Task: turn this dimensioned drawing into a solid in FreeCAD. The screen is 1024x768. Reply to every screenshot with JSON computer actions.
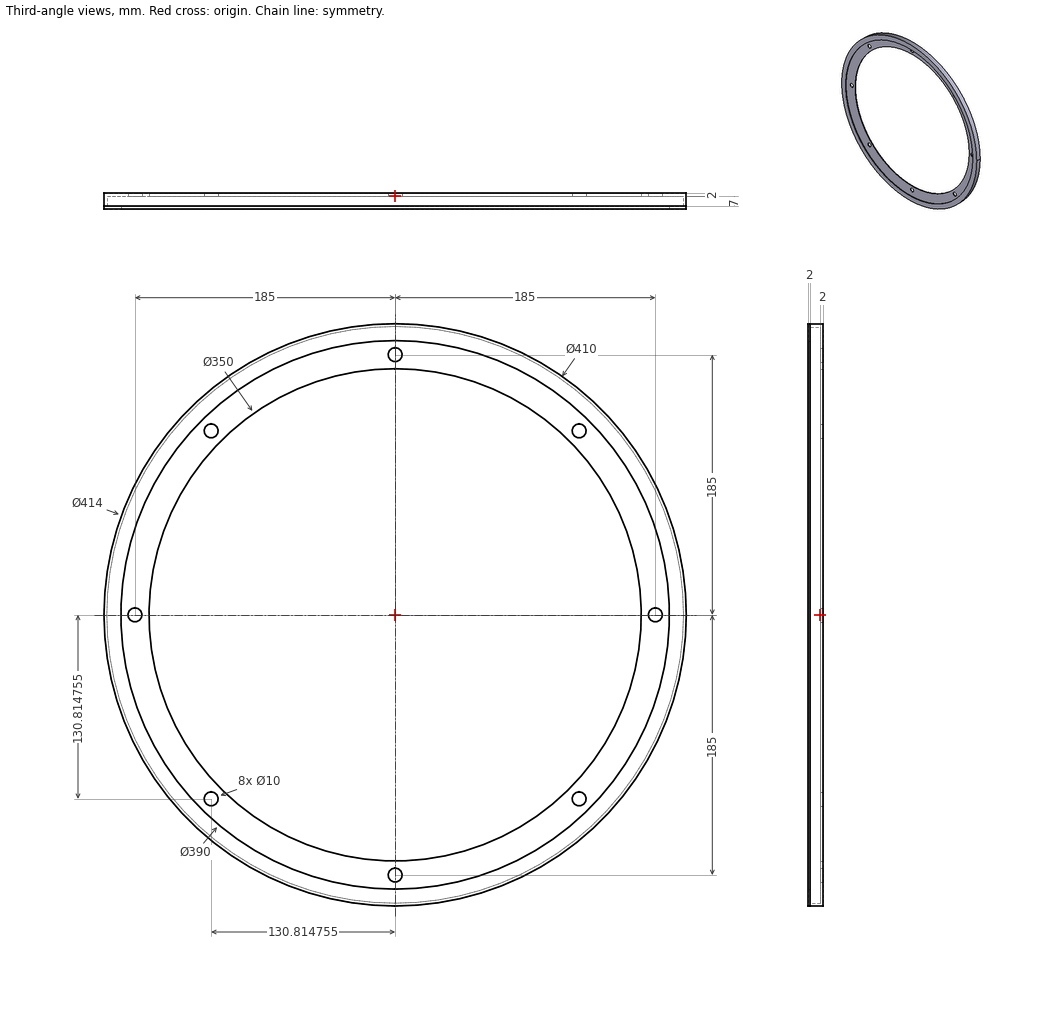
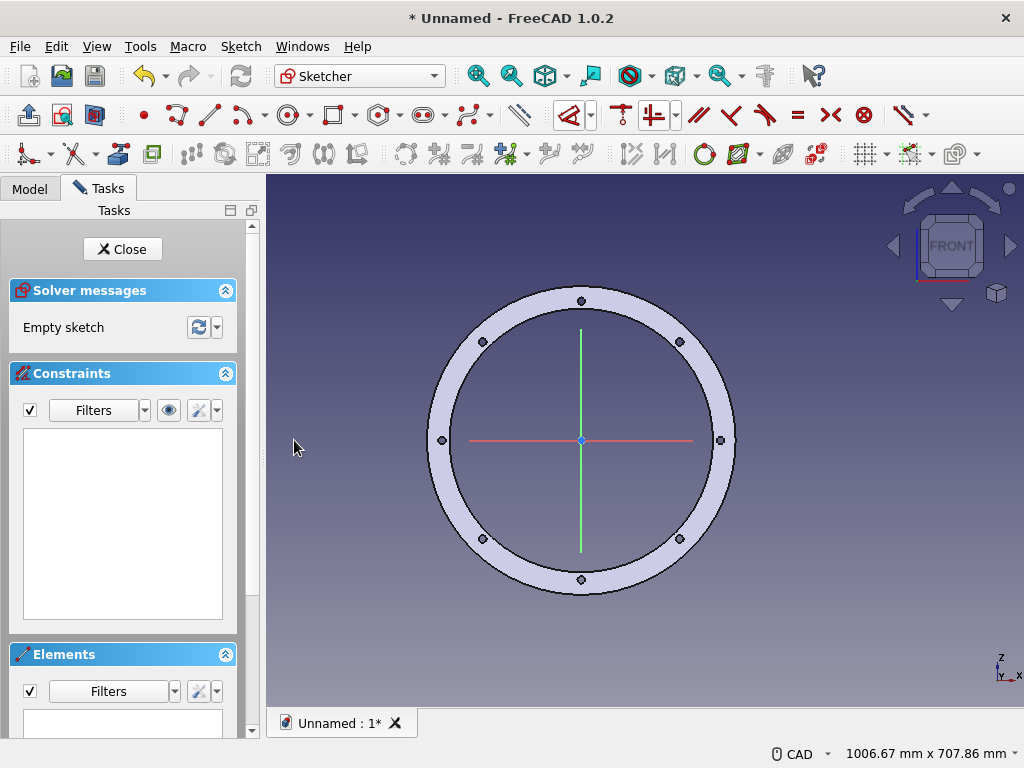
{"action": "left_click", "coordinate": [288, 116]}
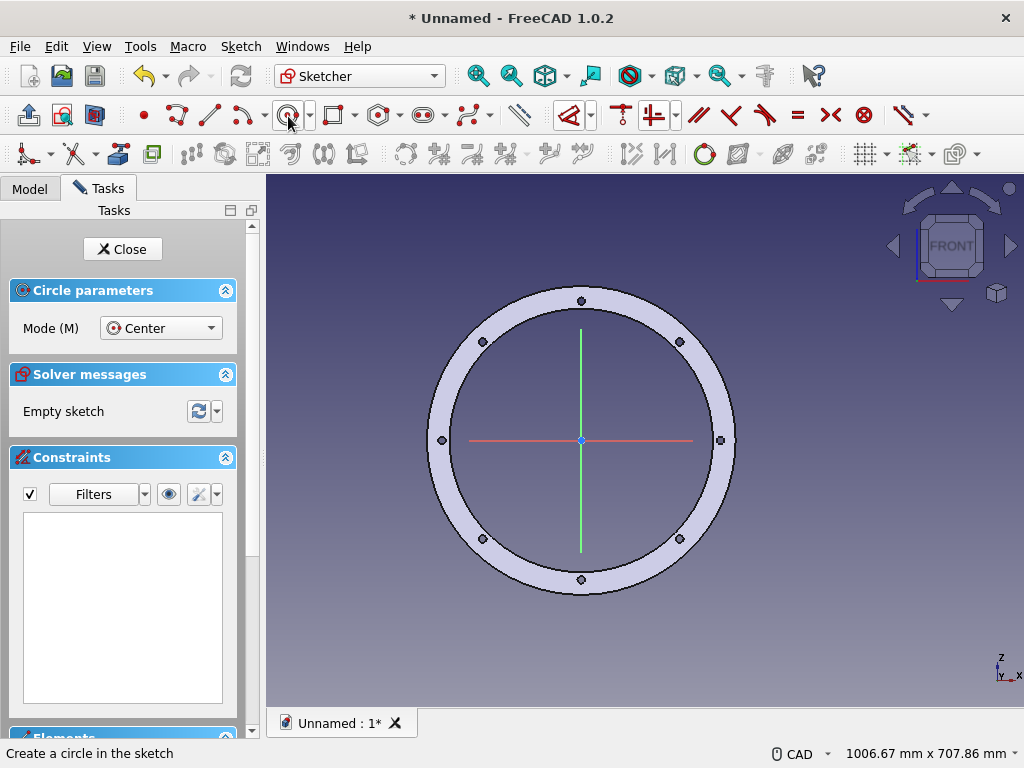
{"action": "left_click", "coordinate": [581, 441]}
{"action": "mouse_move", "coordinate": [691, 330]}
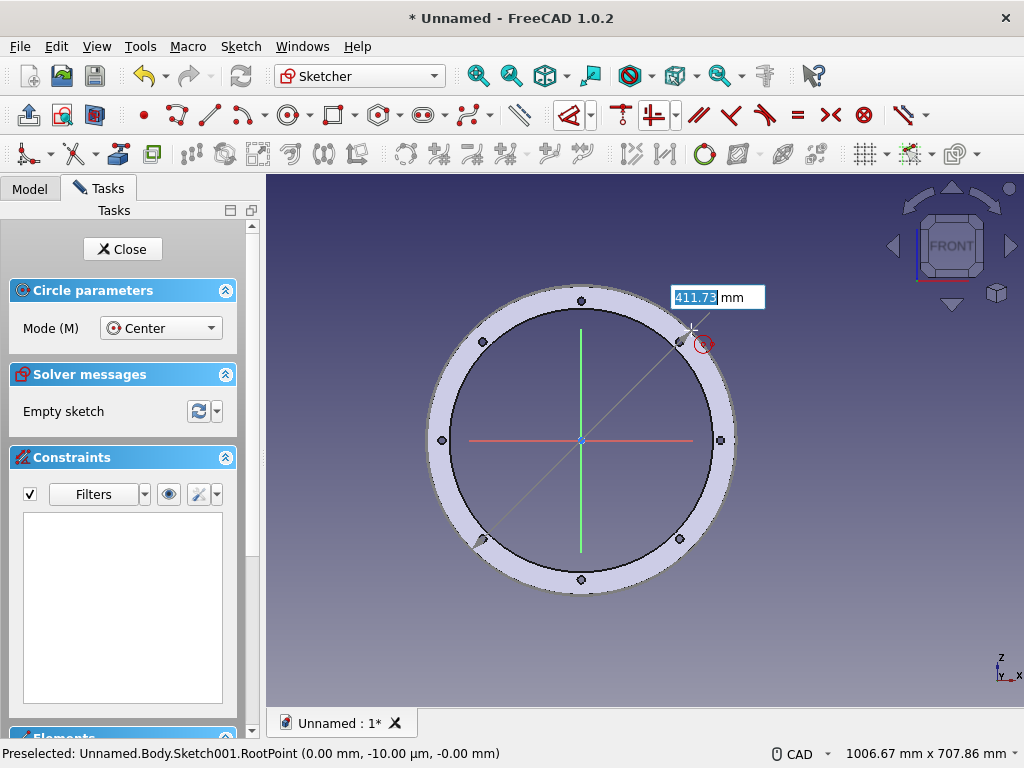
{"action": "type", "text": "414"}
{"action": "key", "text": "Return"}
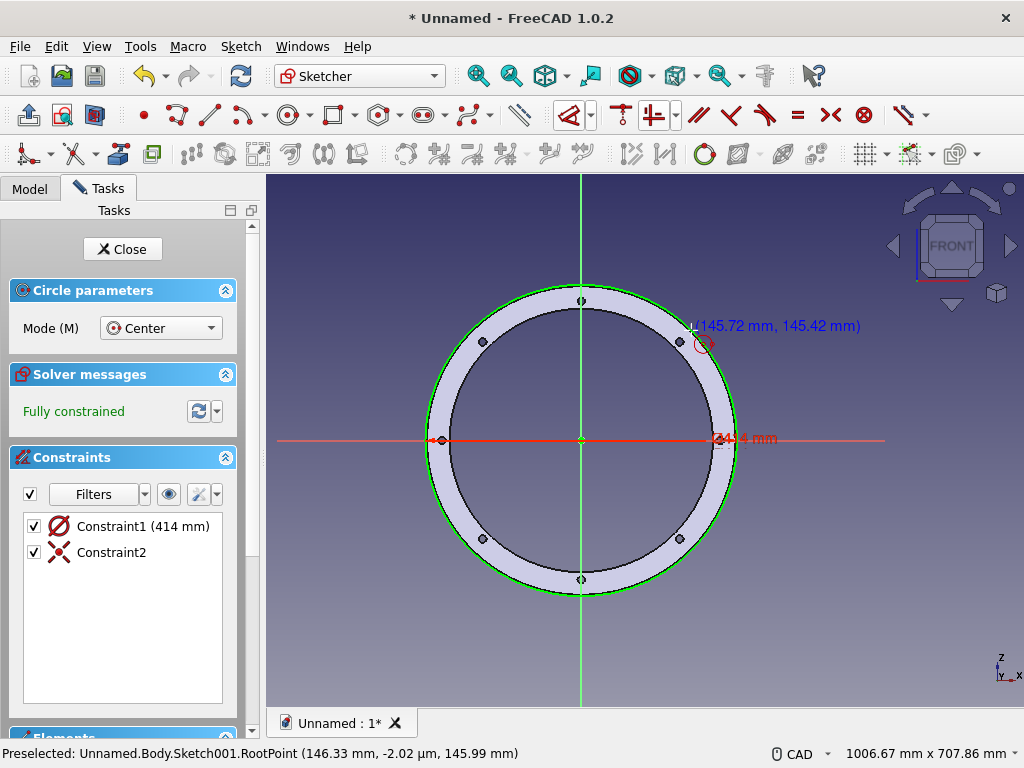
{"action": "left_click", "coordinate": [581, 441]}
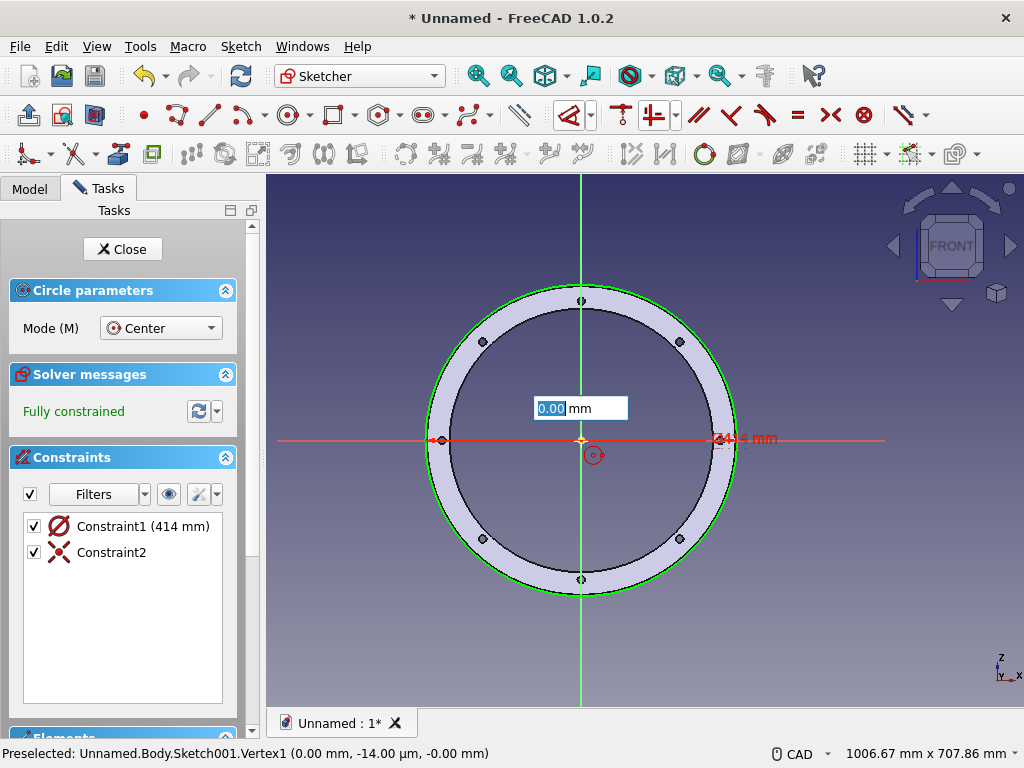
{"action": "scroll", "coordinate": [528, 586], "scroll_direction": "up", "scroll_amount": 12}
{"action": "mouse_move", "coordinate": [530, 573]}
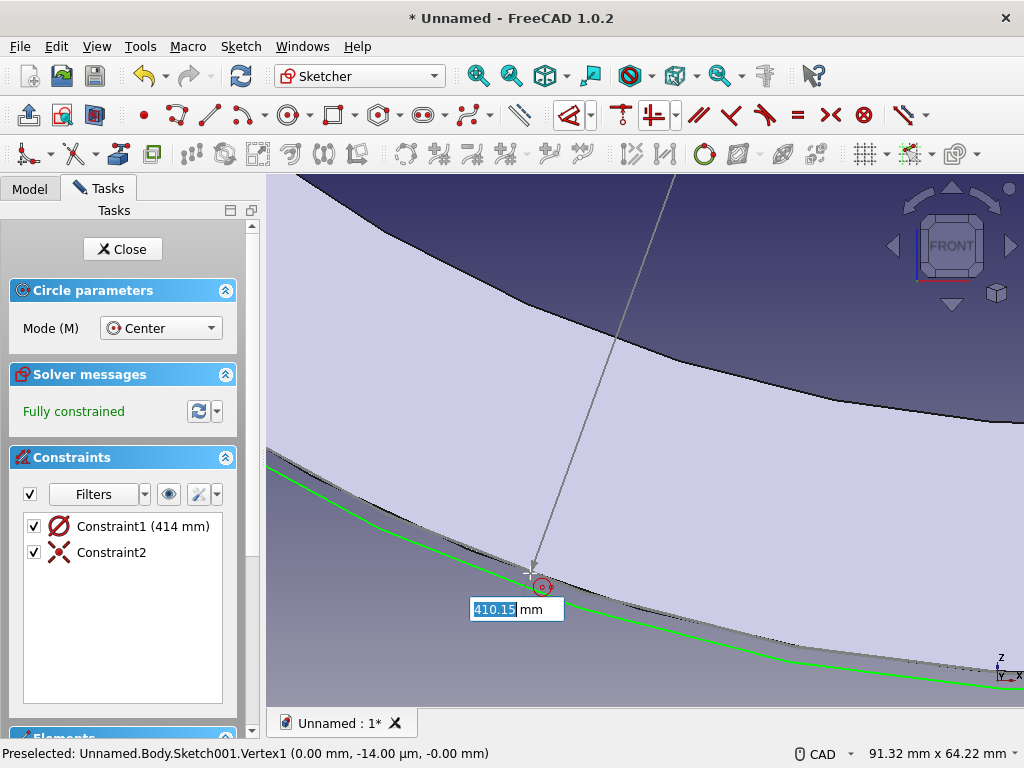
{"action": "type", "text": "410"}
{"action": "key", "text": "Return"}
{"action": "key", "text": "Escape"}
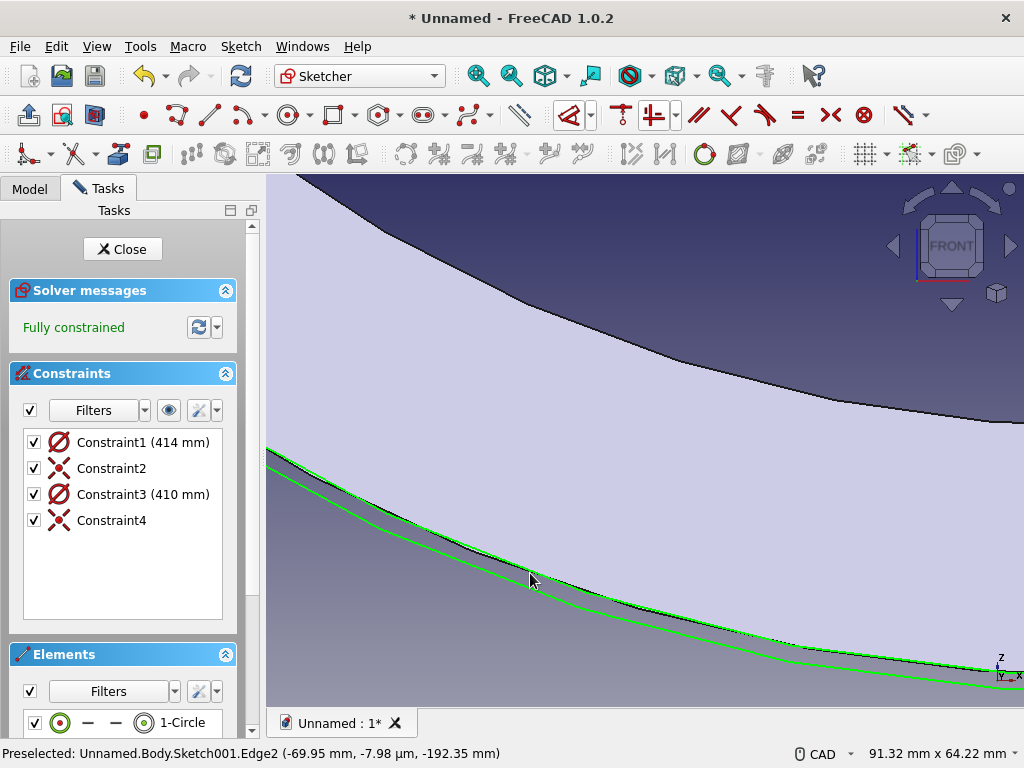
{"action": "left_click", "coordinate": [123, 249]}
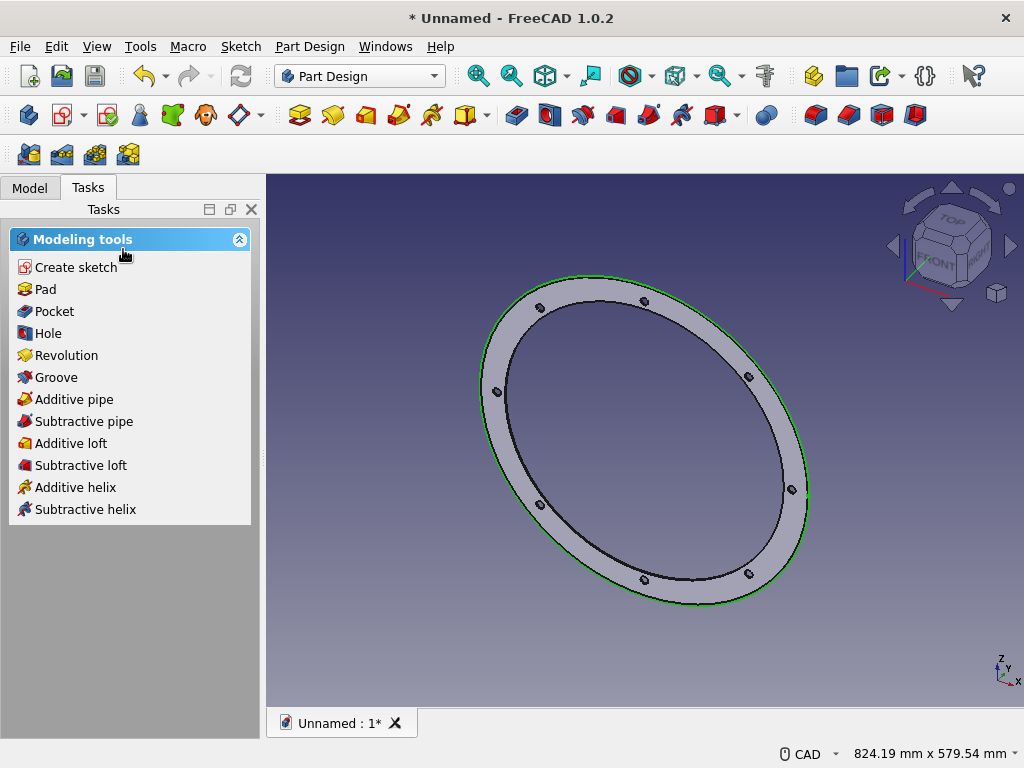
{"action": "left_click", "coordinate": [300, 116]}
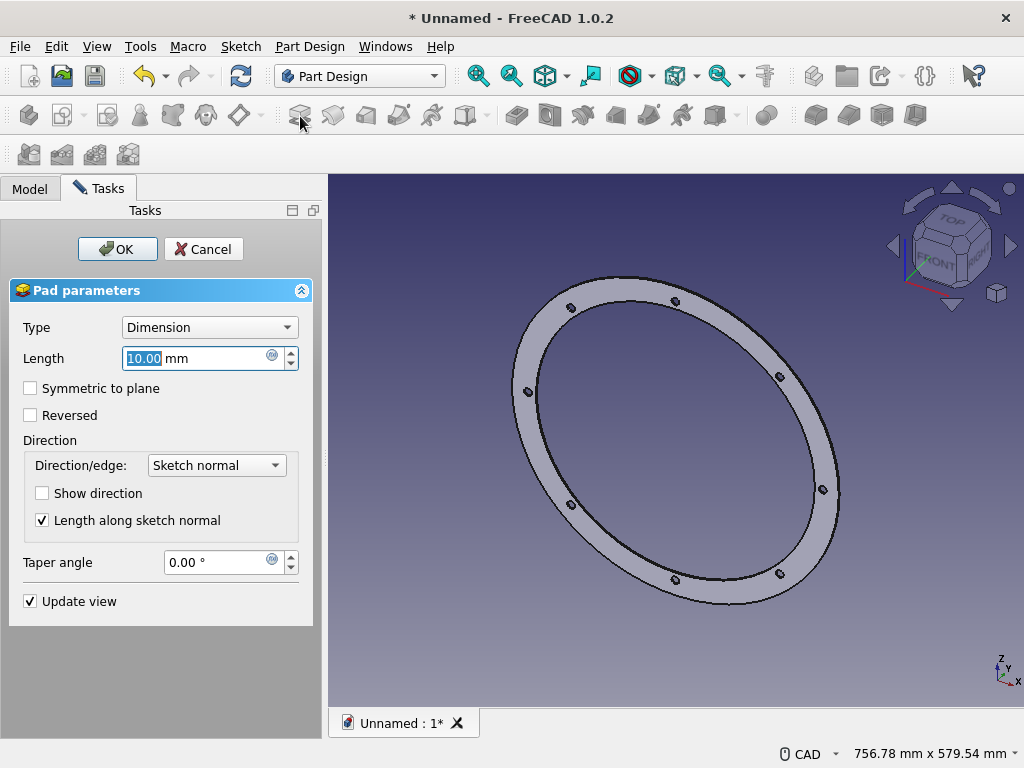
{"action": "left_click", "coordinate": [210, 328]}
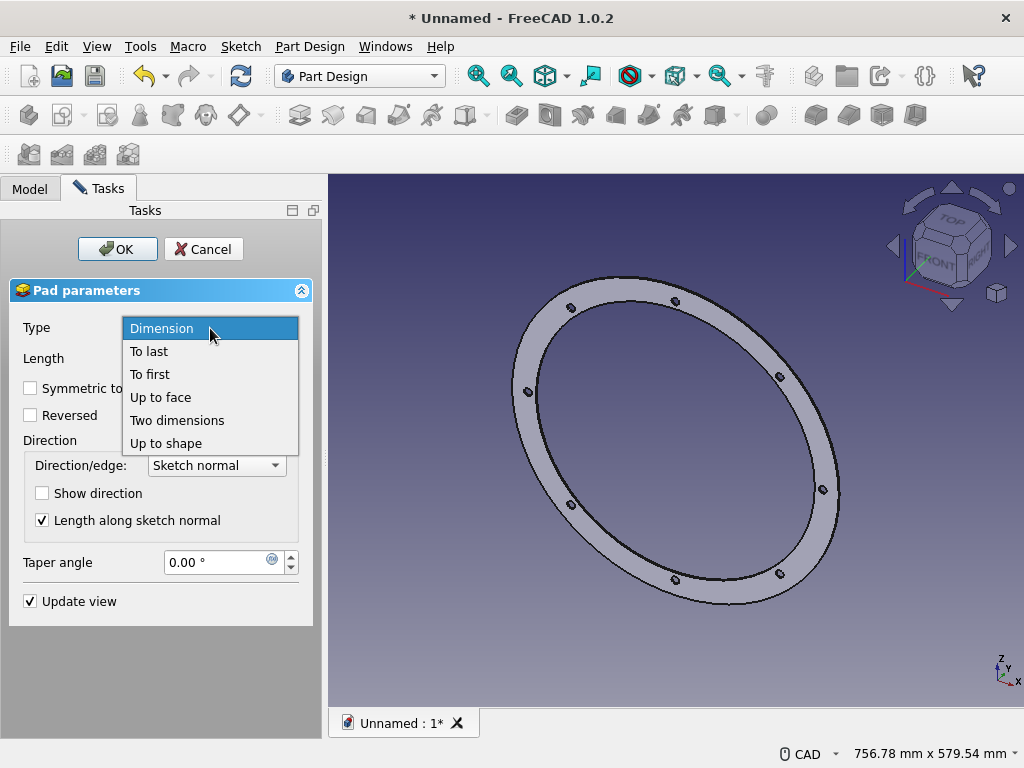
{"action": "left_click", "coordinate": [208, 420]}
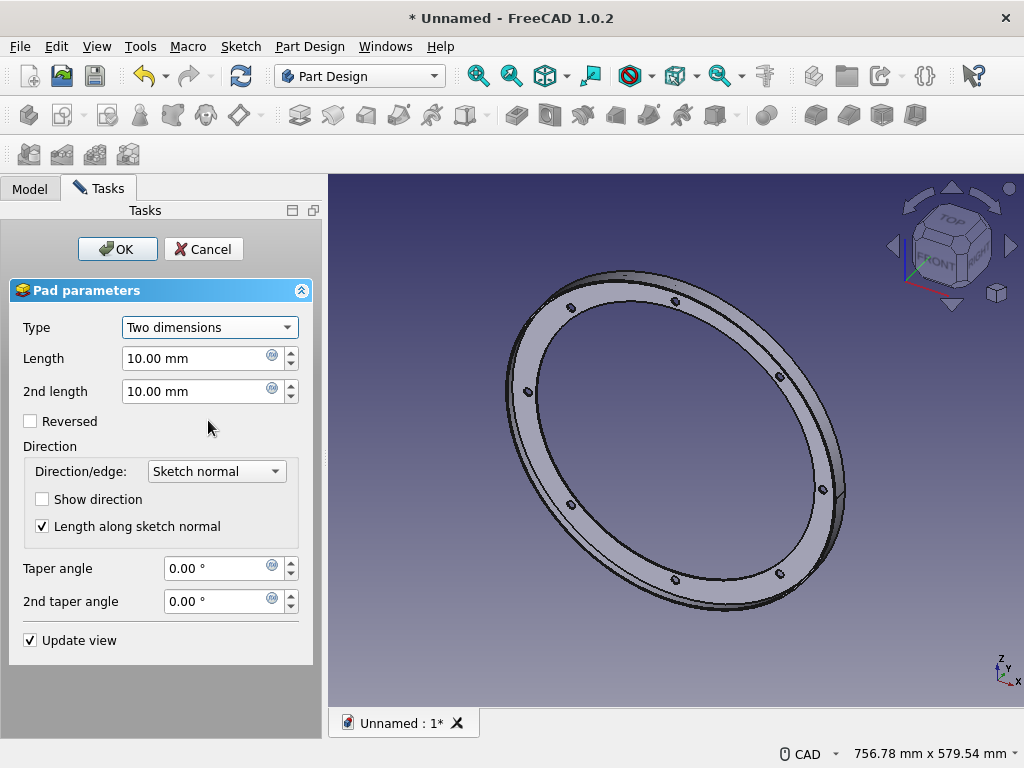
{"action": "triple_click", "coordinate": [204, 358]}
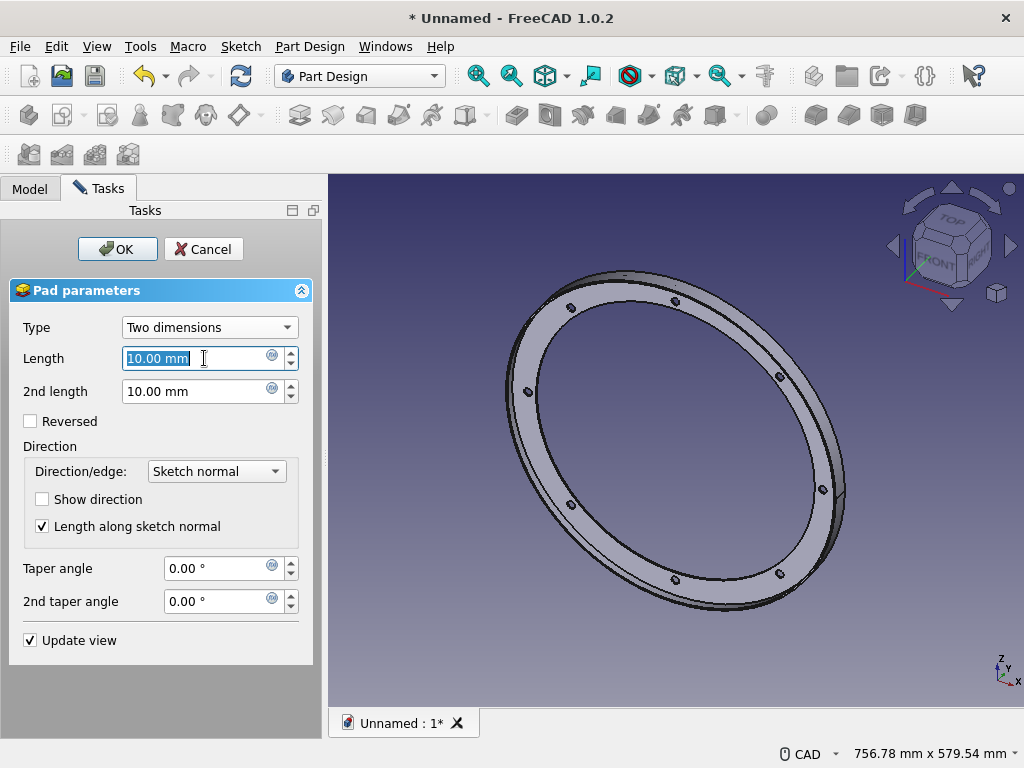
{"action": "type", "text": "7"}
{"action": "key", "text": "Tab"}